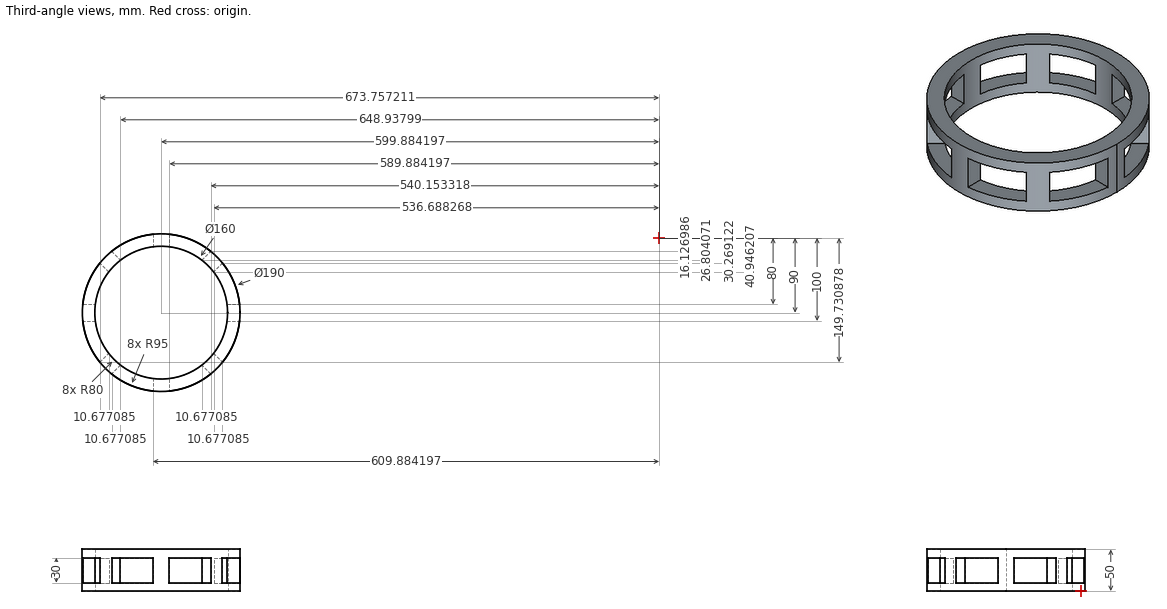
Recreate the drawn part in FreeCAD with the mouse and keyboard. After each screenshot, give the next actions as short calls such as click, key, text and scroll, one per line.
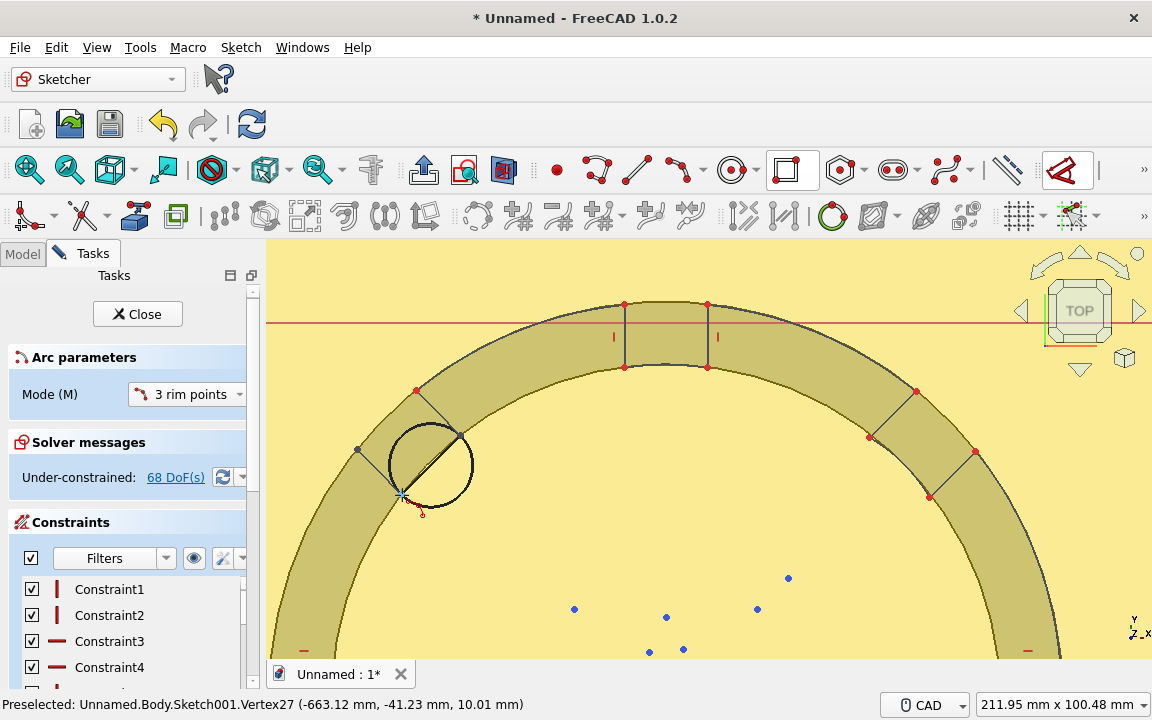
scroll(429, 462, up, 10)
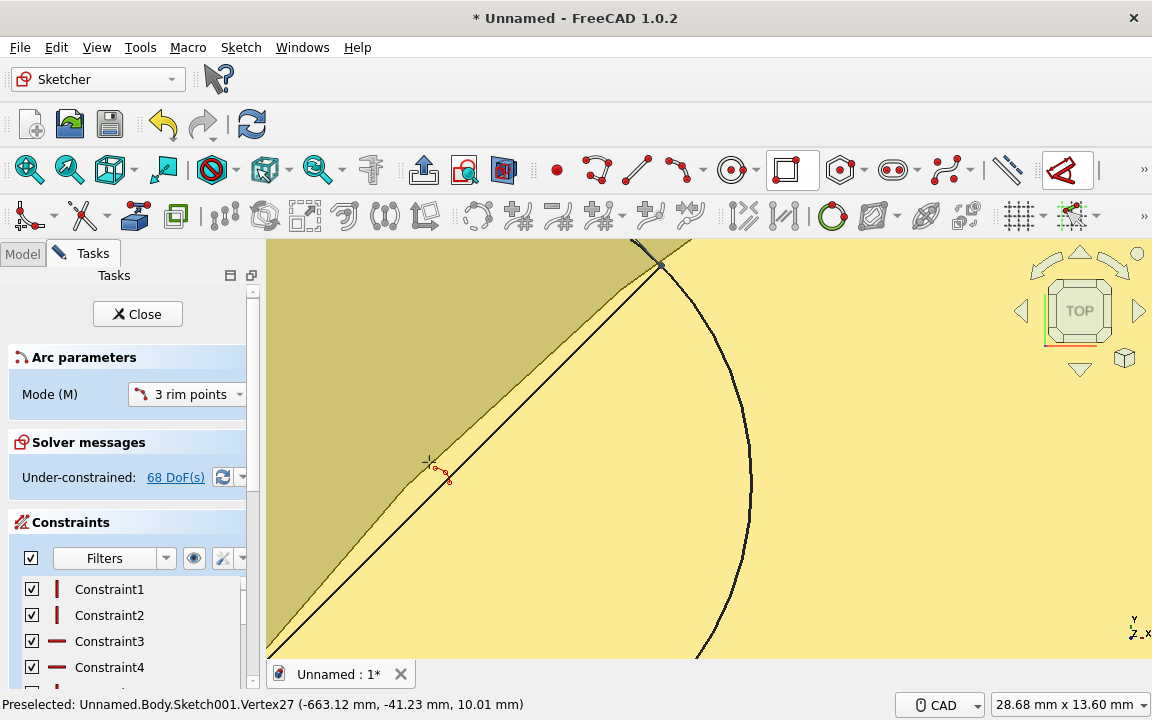
click(431, 461)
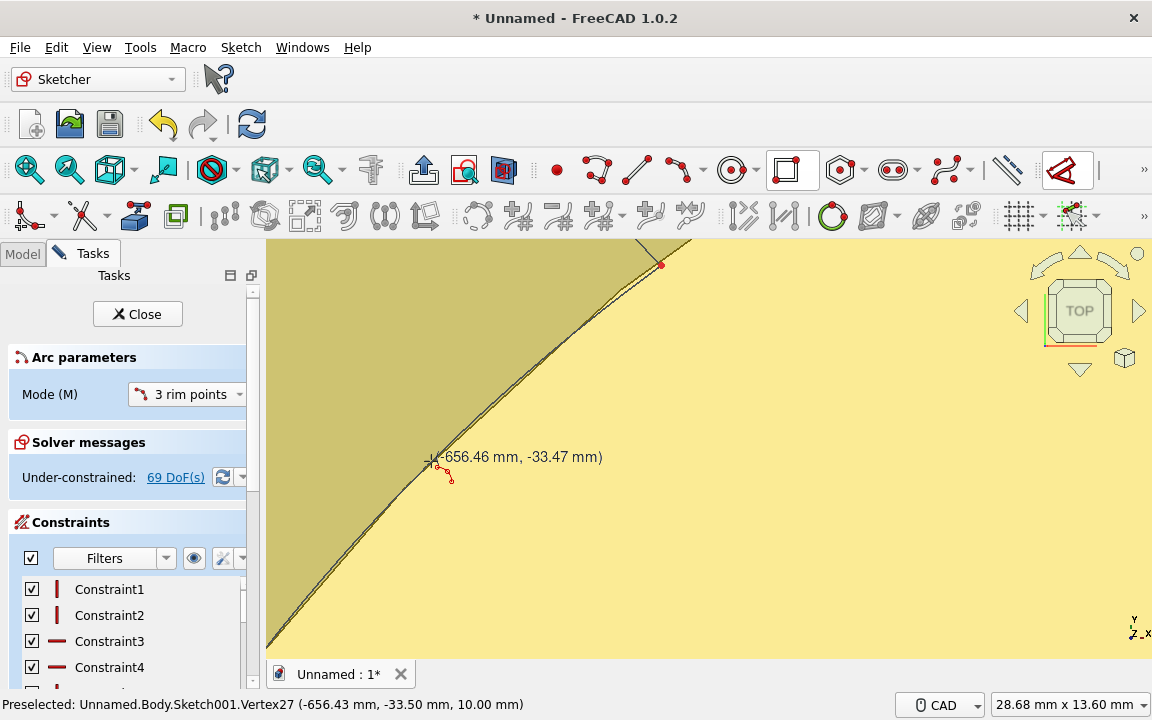
scroll(560, 357, down, 15)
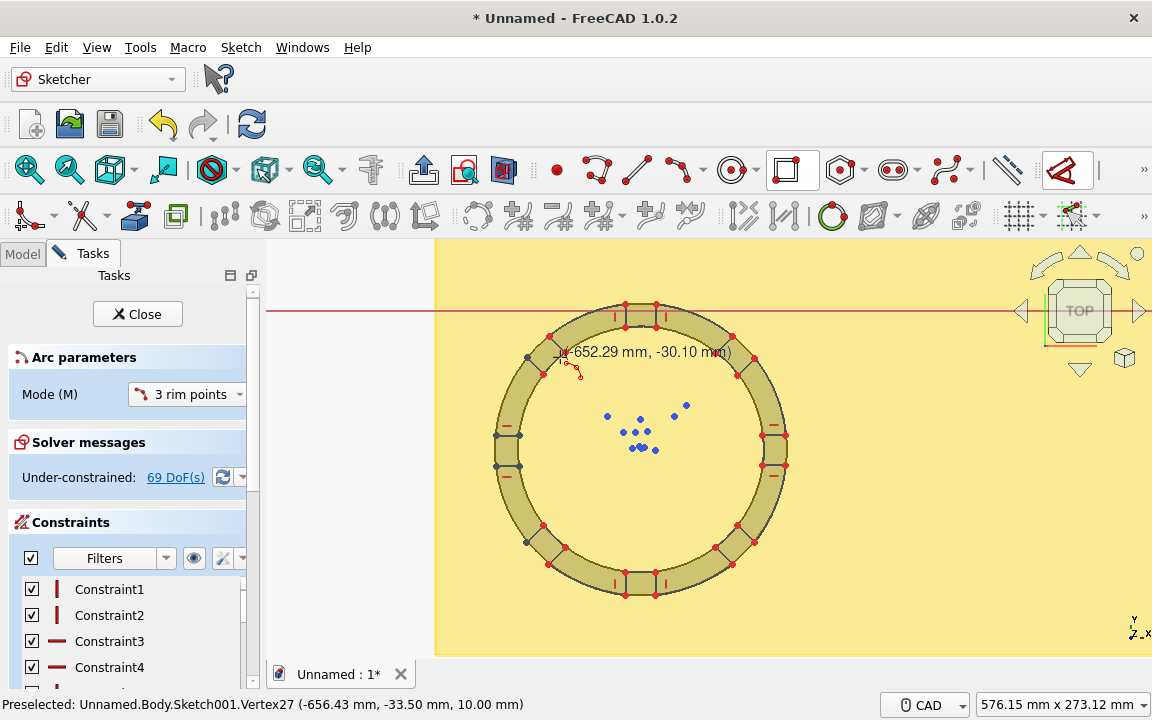
scroll(527, 358, up, 2)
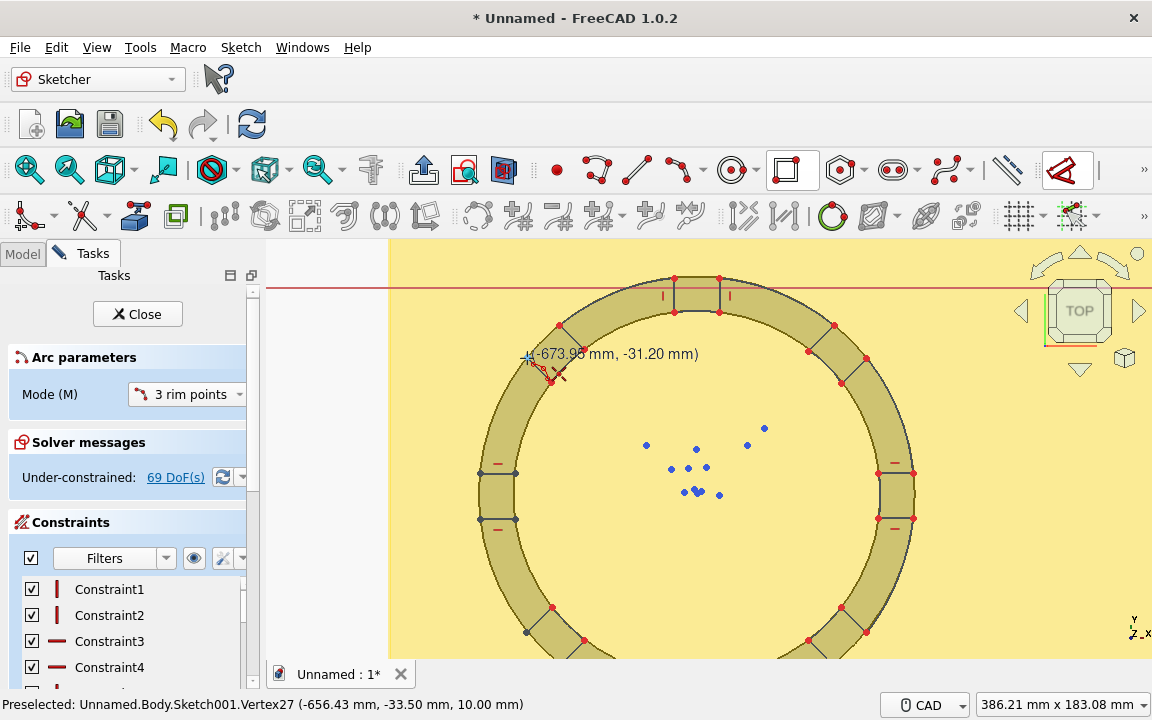
click(528, 358)
click(481, 474)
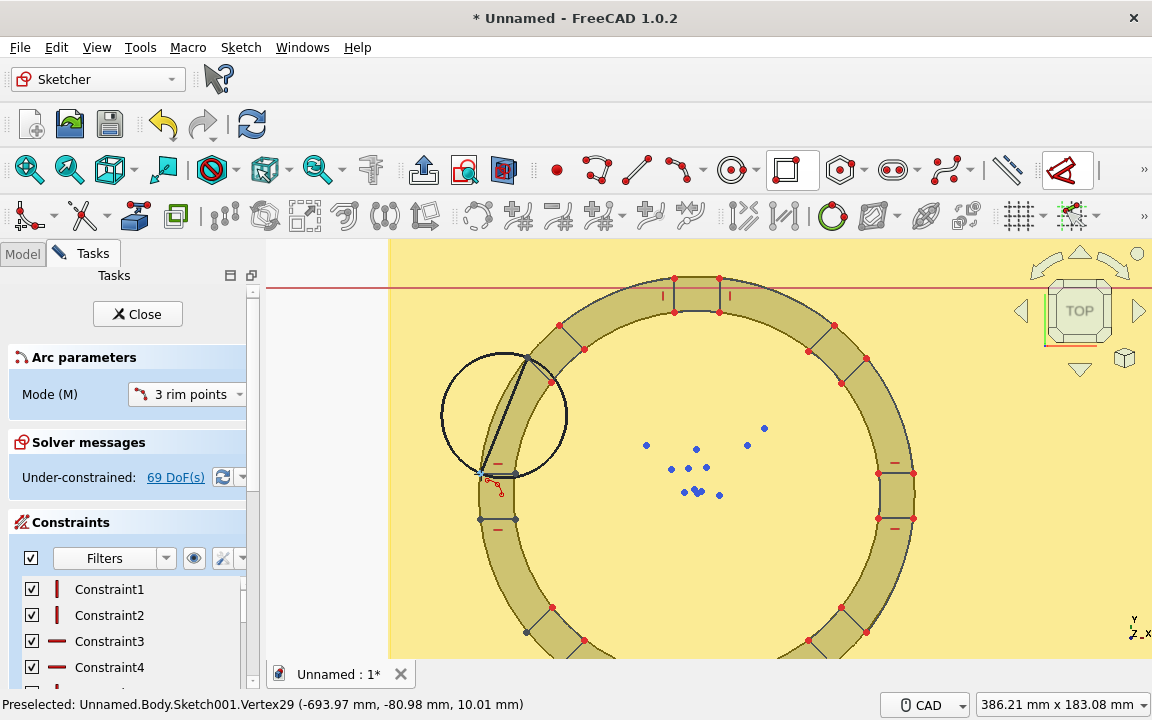
scroll(495, 411, up, 3)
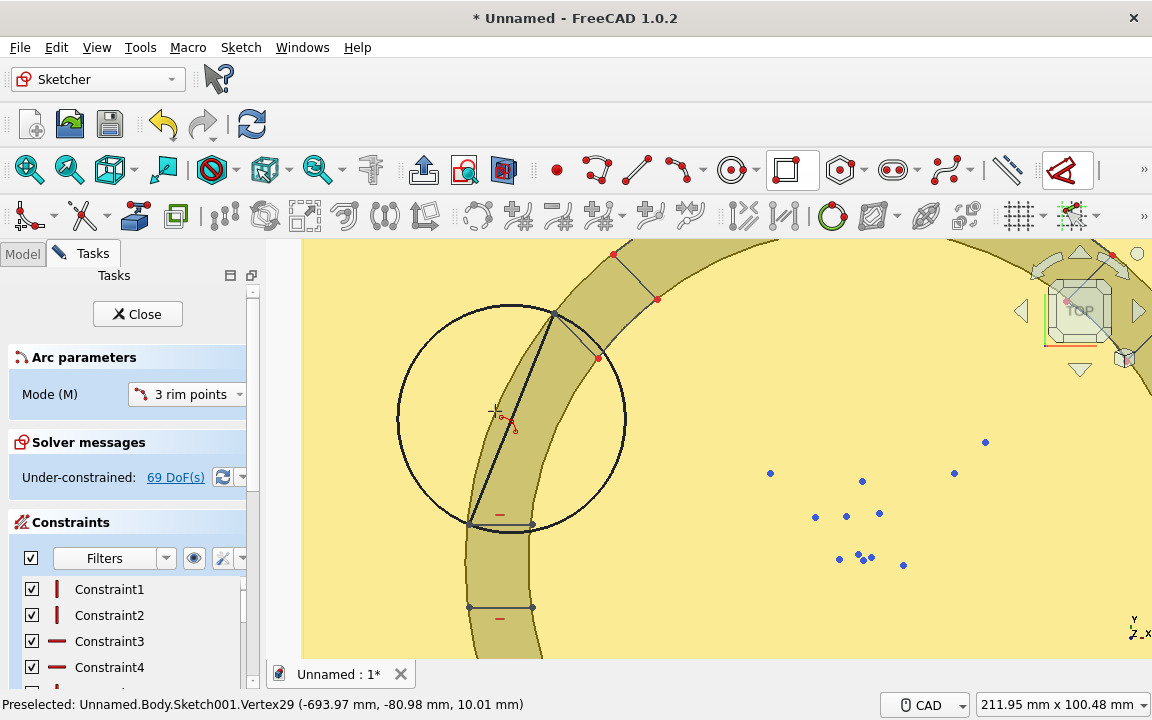
click(496, 410)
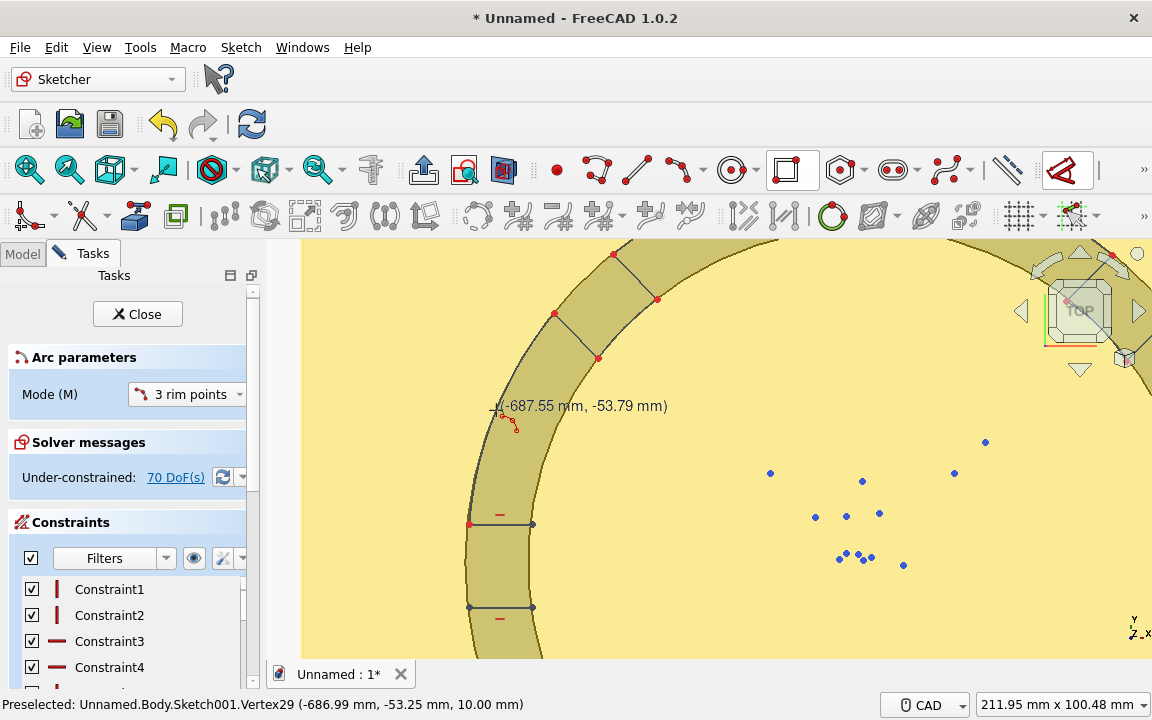
click(532, 525)
click(532, 608)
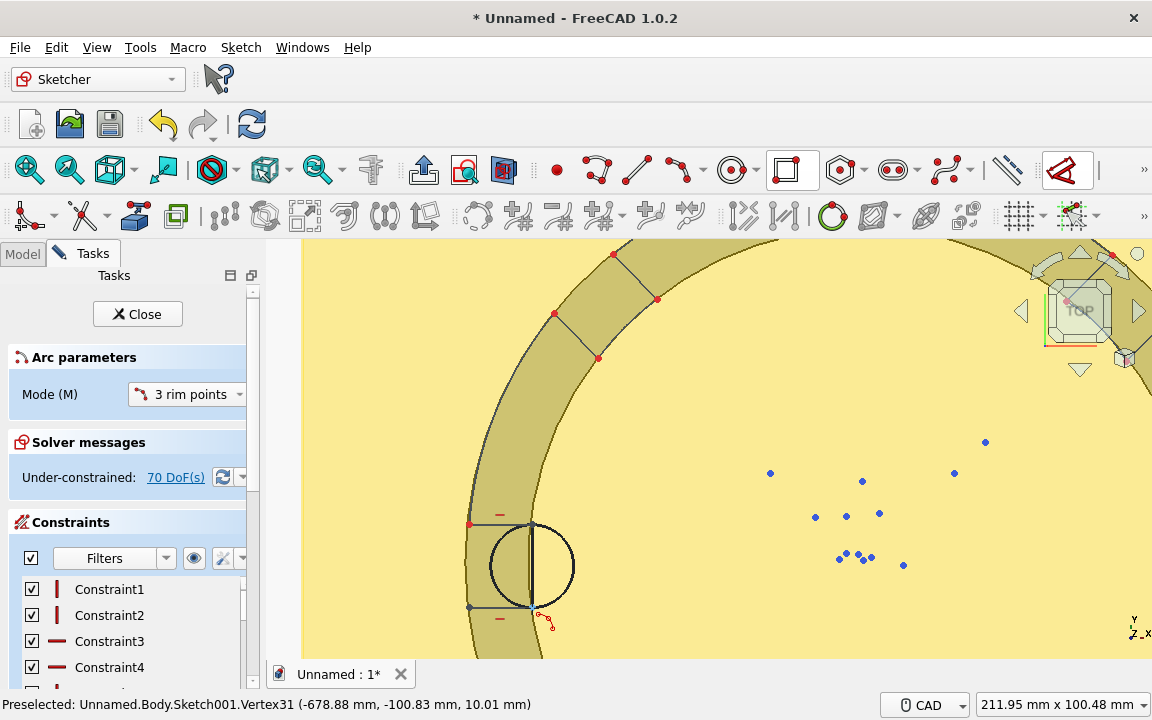
scroll(528, 562, up, 10)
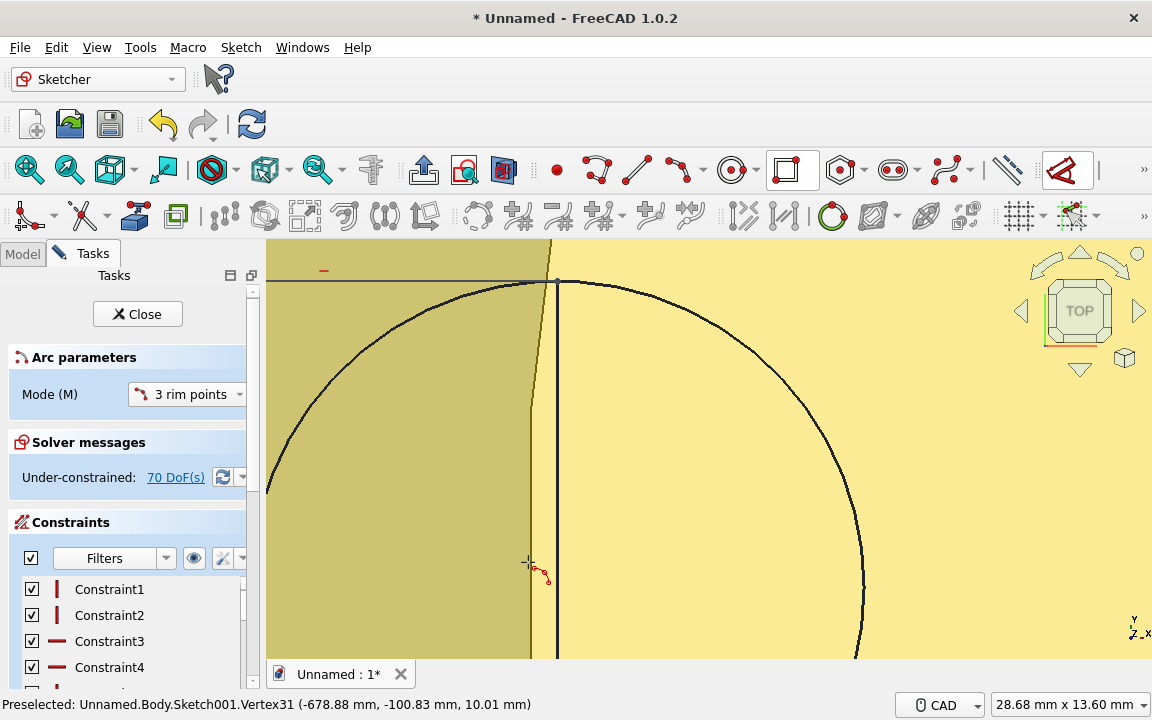
click(526, 560)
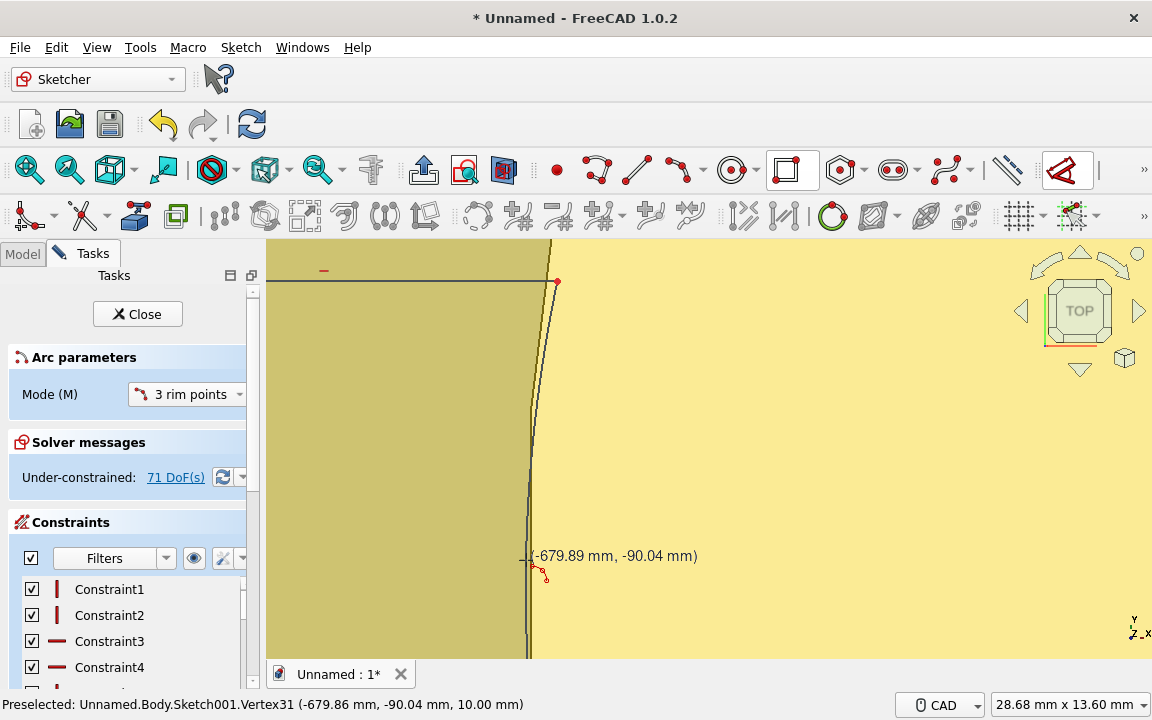
scroll(517, 443, down, 15)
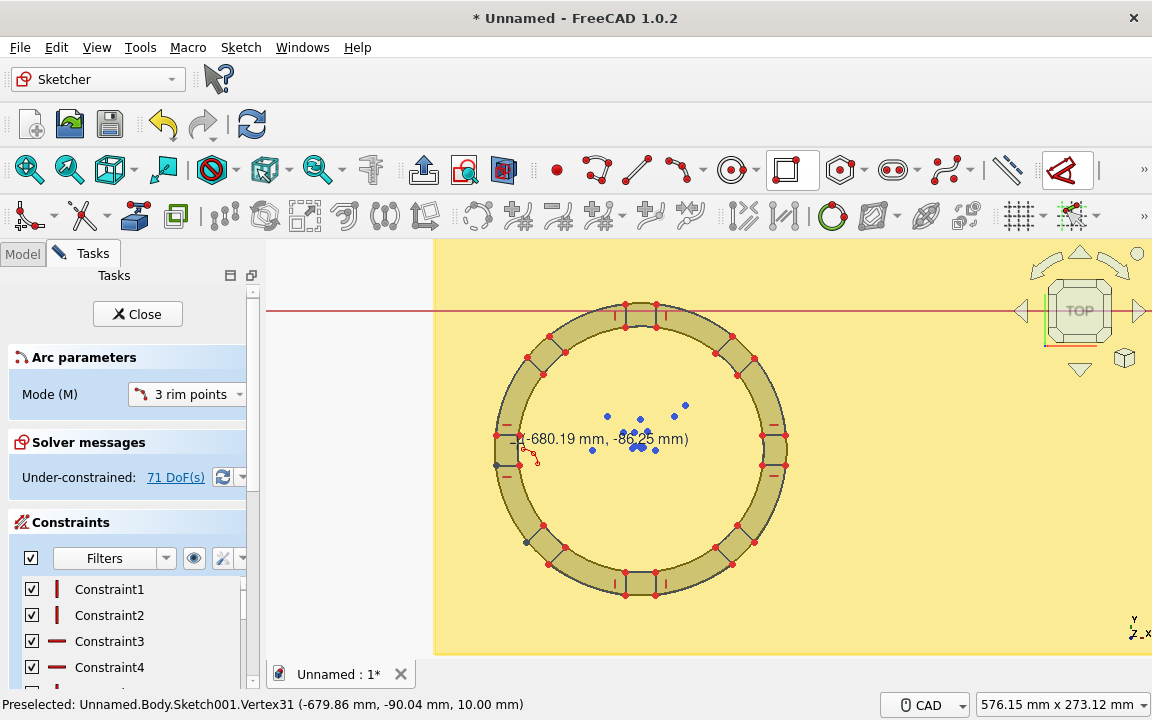
scroll(495, 465, up, 2)